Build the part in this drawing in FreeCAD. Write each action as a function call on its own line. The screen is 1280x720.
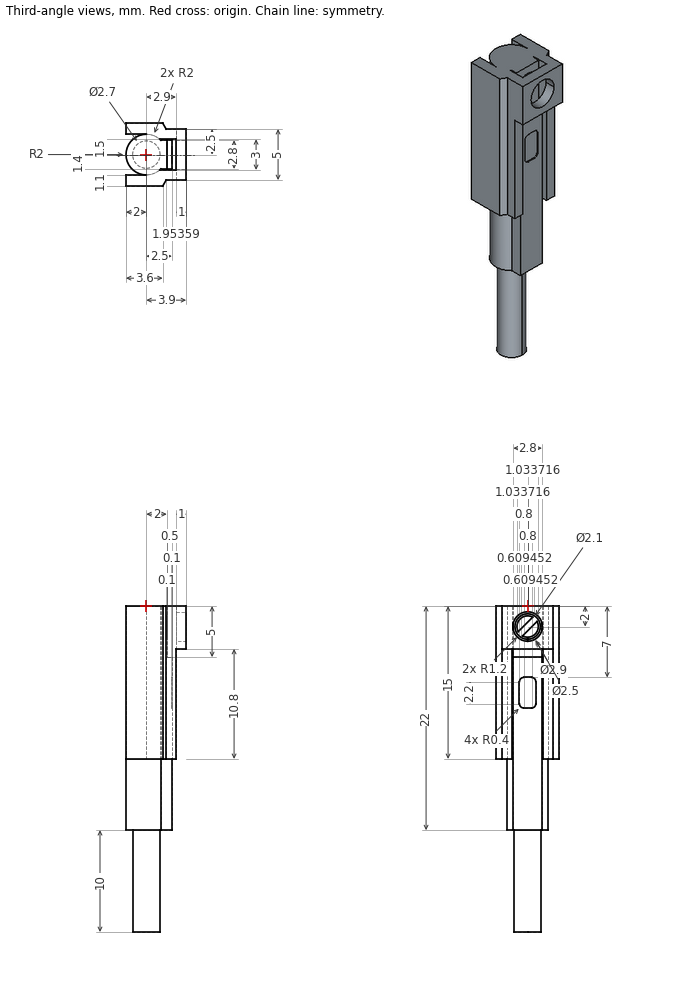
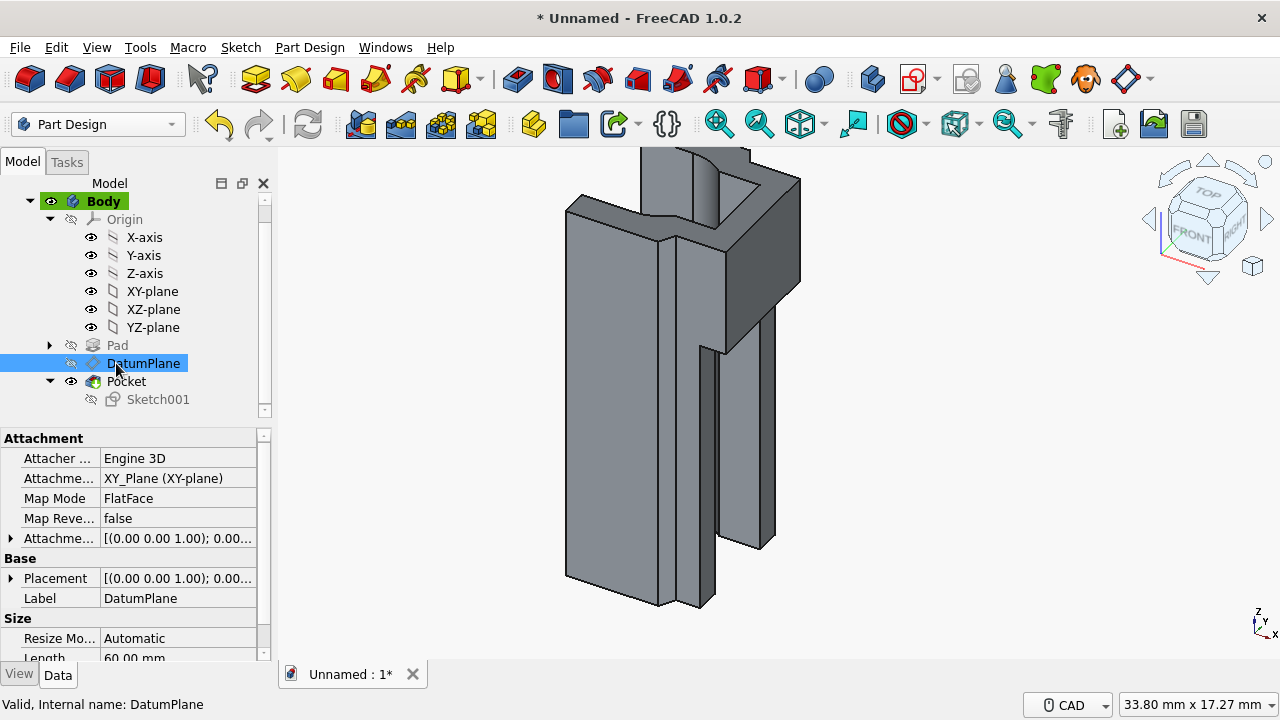
click(720, 124)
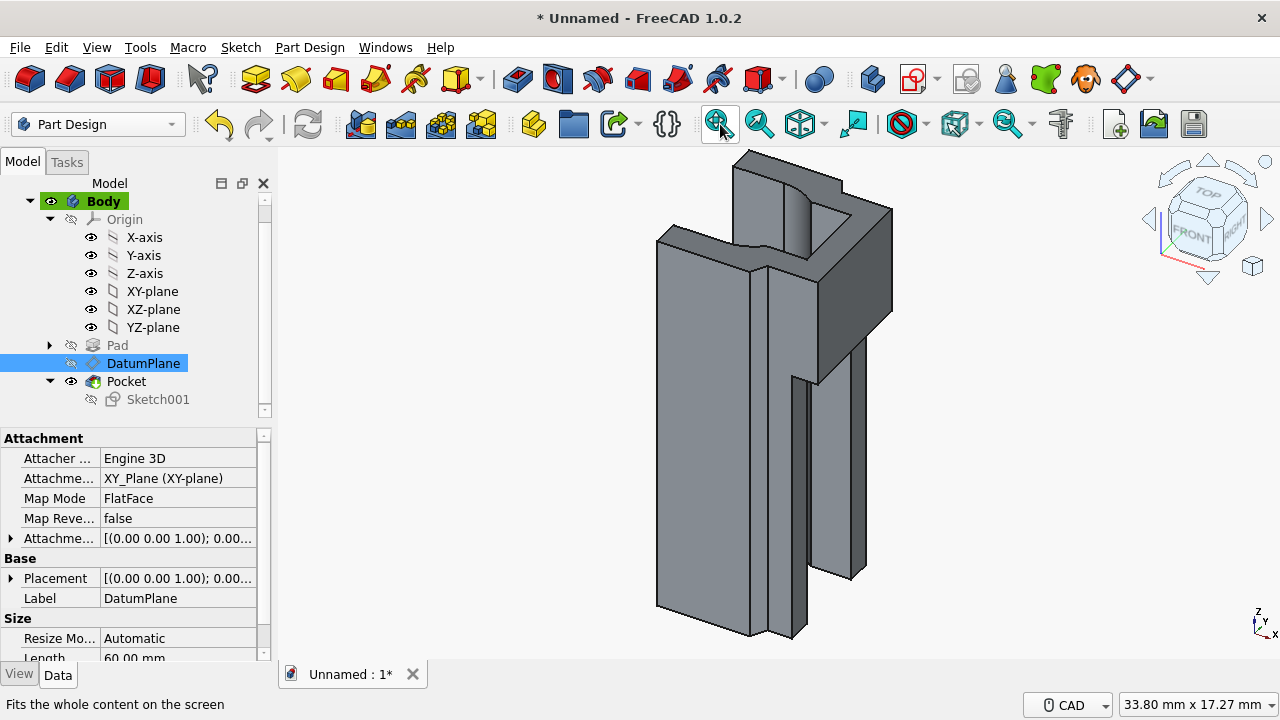
click(855, 296)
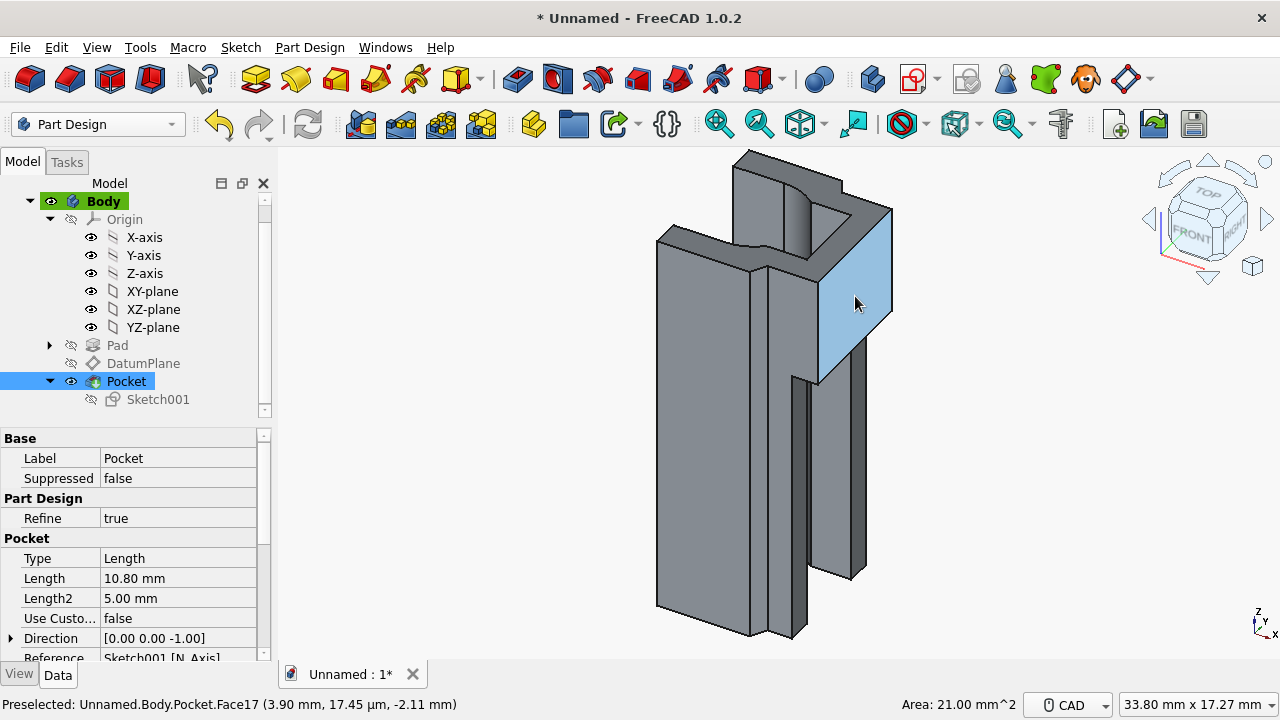
click(914, 80)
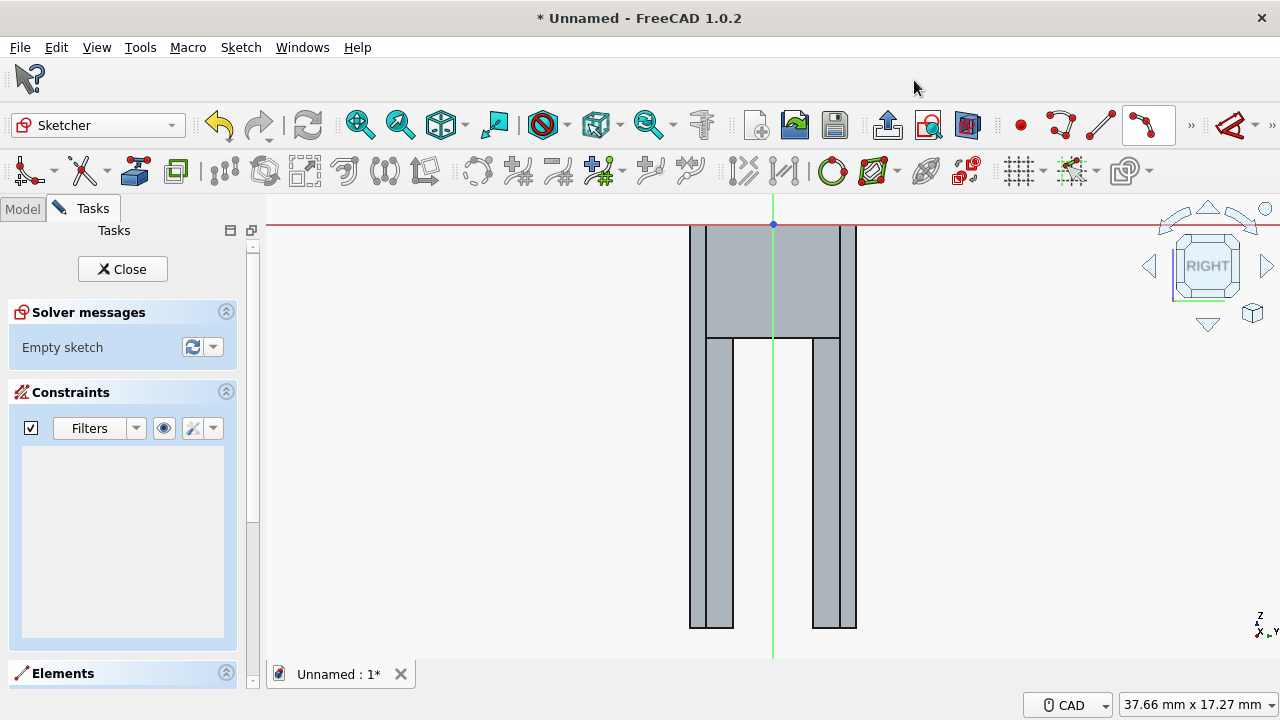
scroll(704, 426, down, 5)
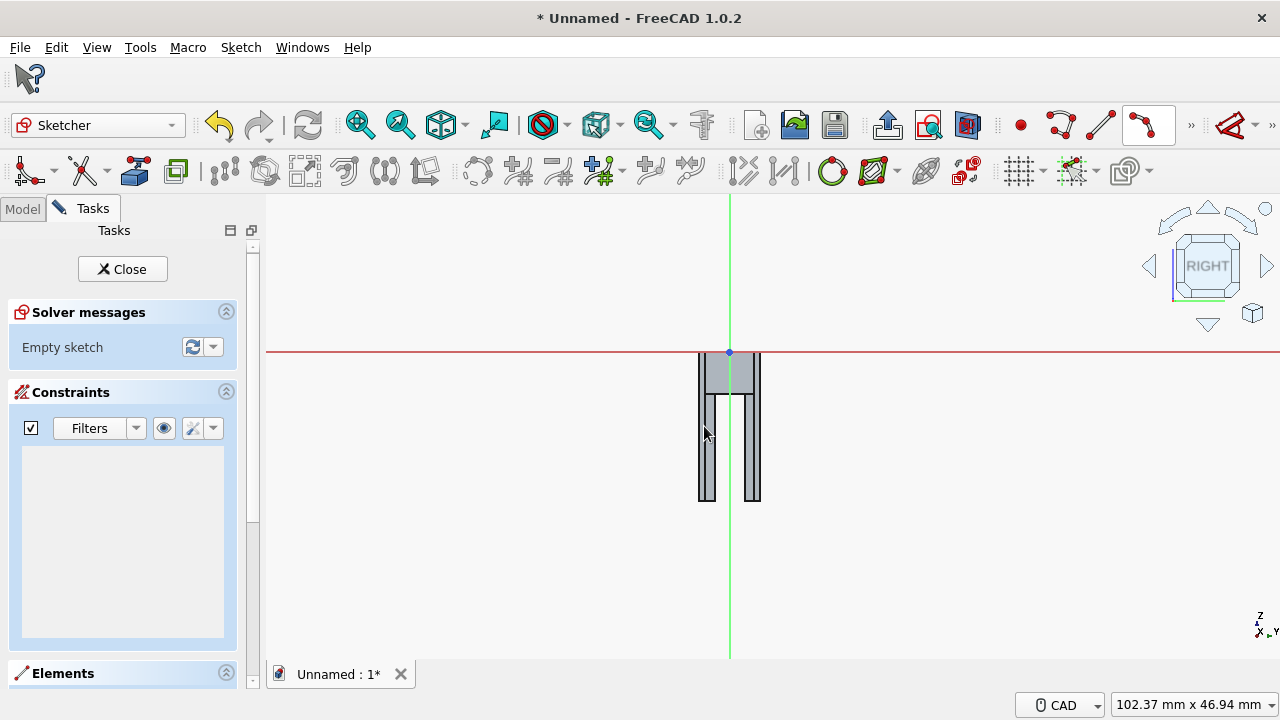
scroll(733, 362, up, 11)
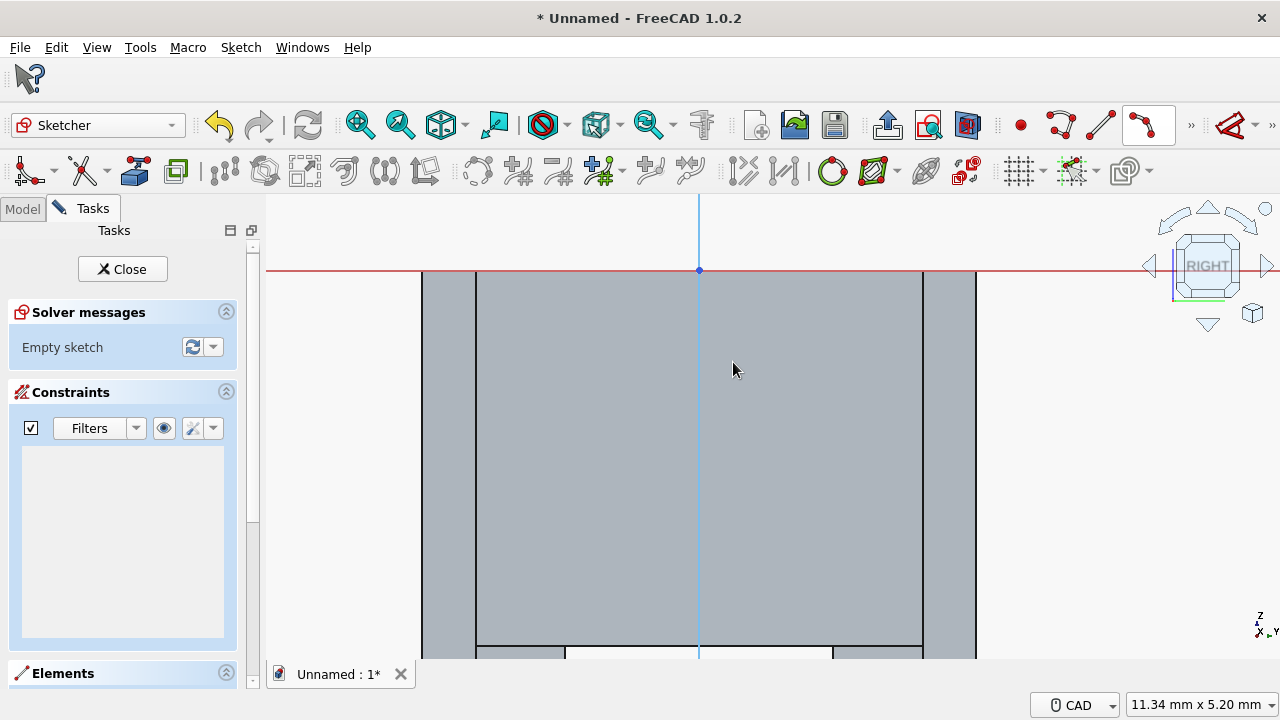
key(g)
key(c)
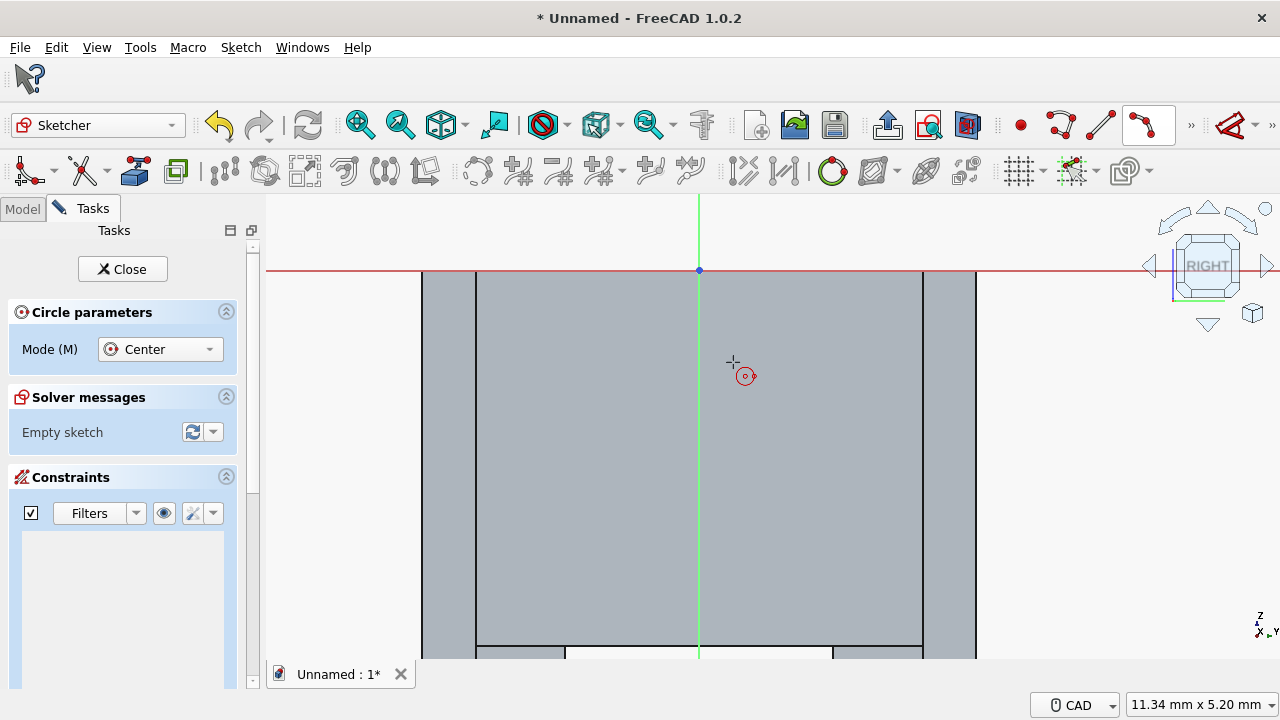
click(699, 450)
click(791, 358)
key(Escape)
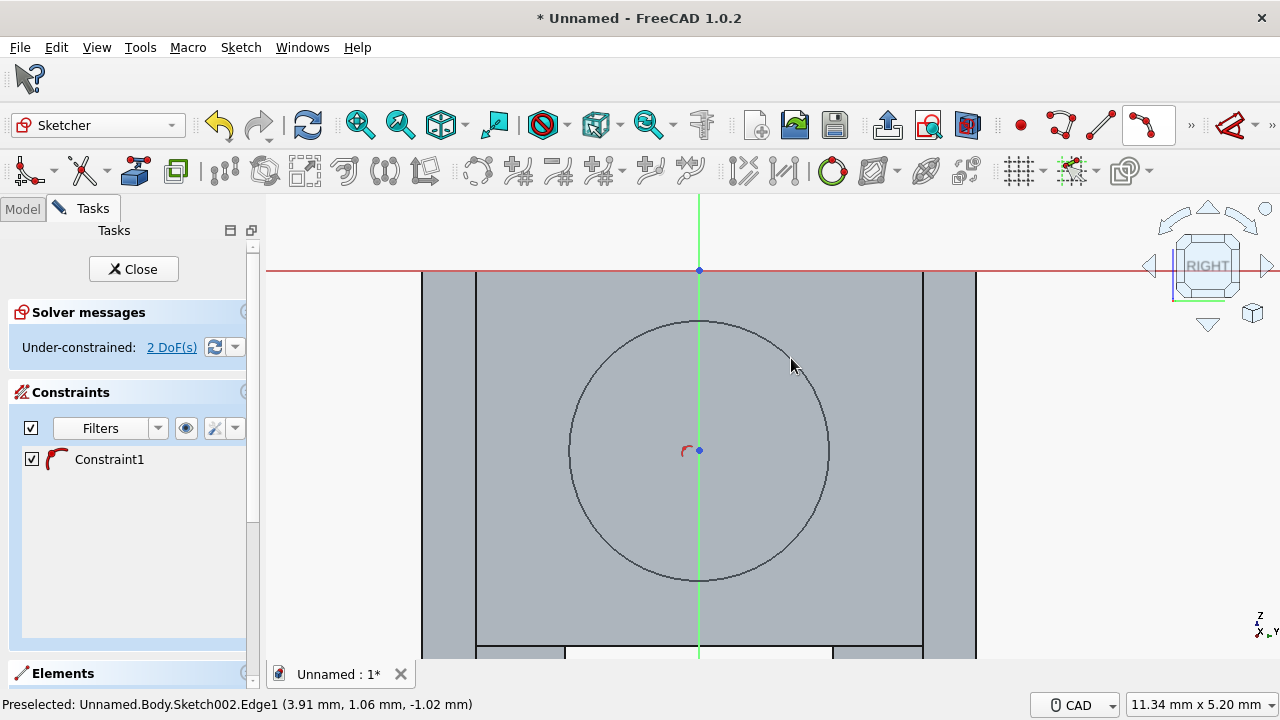
click(1230, 126)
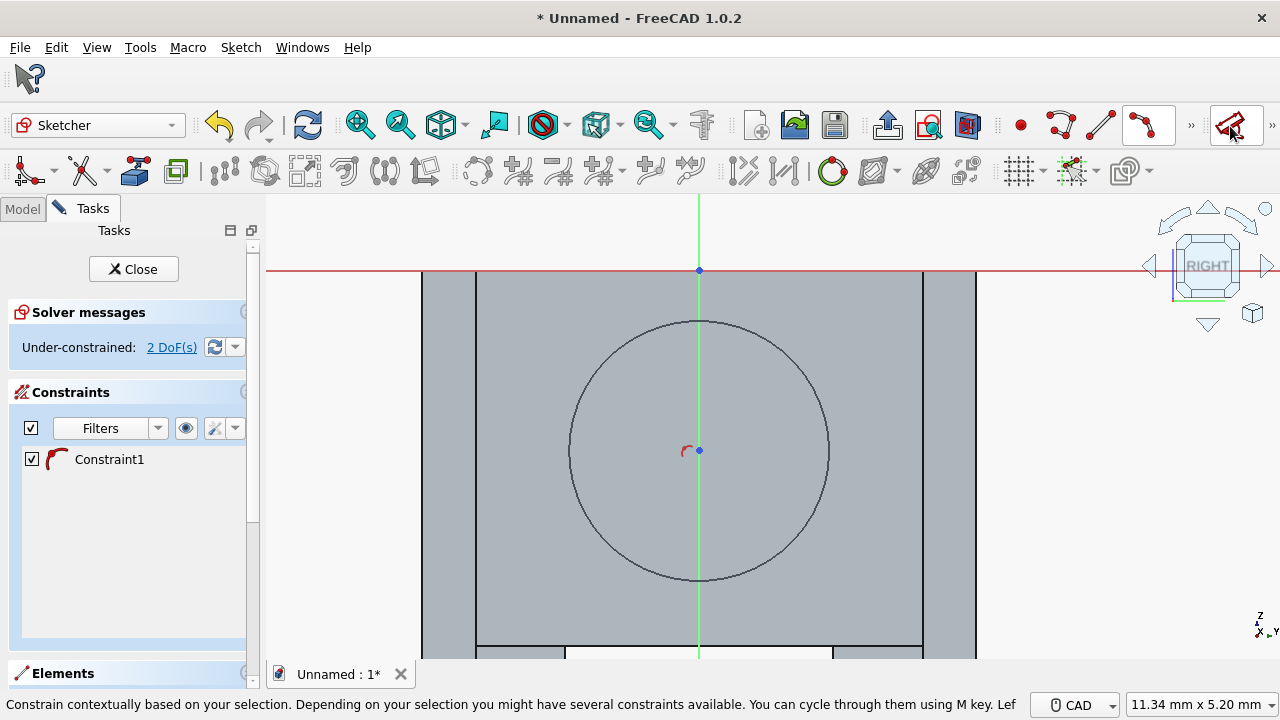
click(791, 359)
click(814, 336)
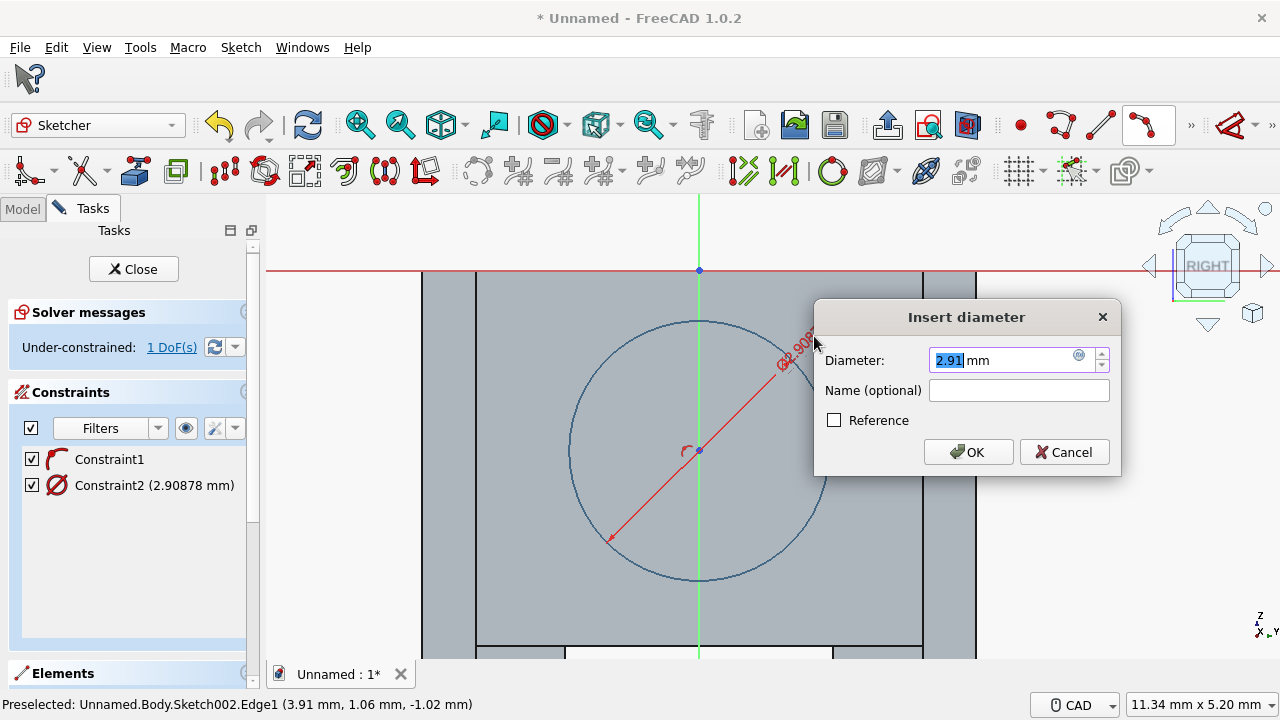
text(2.9)
key(Return)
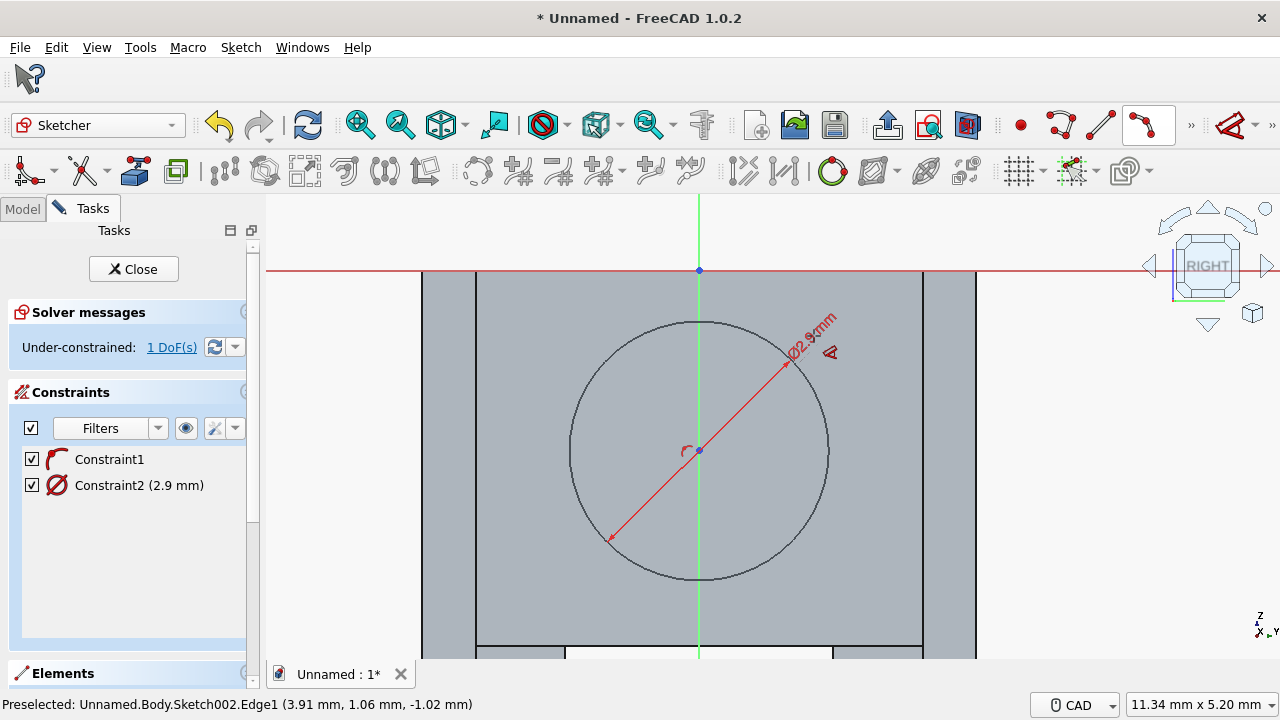
click(699, 451)
click(733, 361)